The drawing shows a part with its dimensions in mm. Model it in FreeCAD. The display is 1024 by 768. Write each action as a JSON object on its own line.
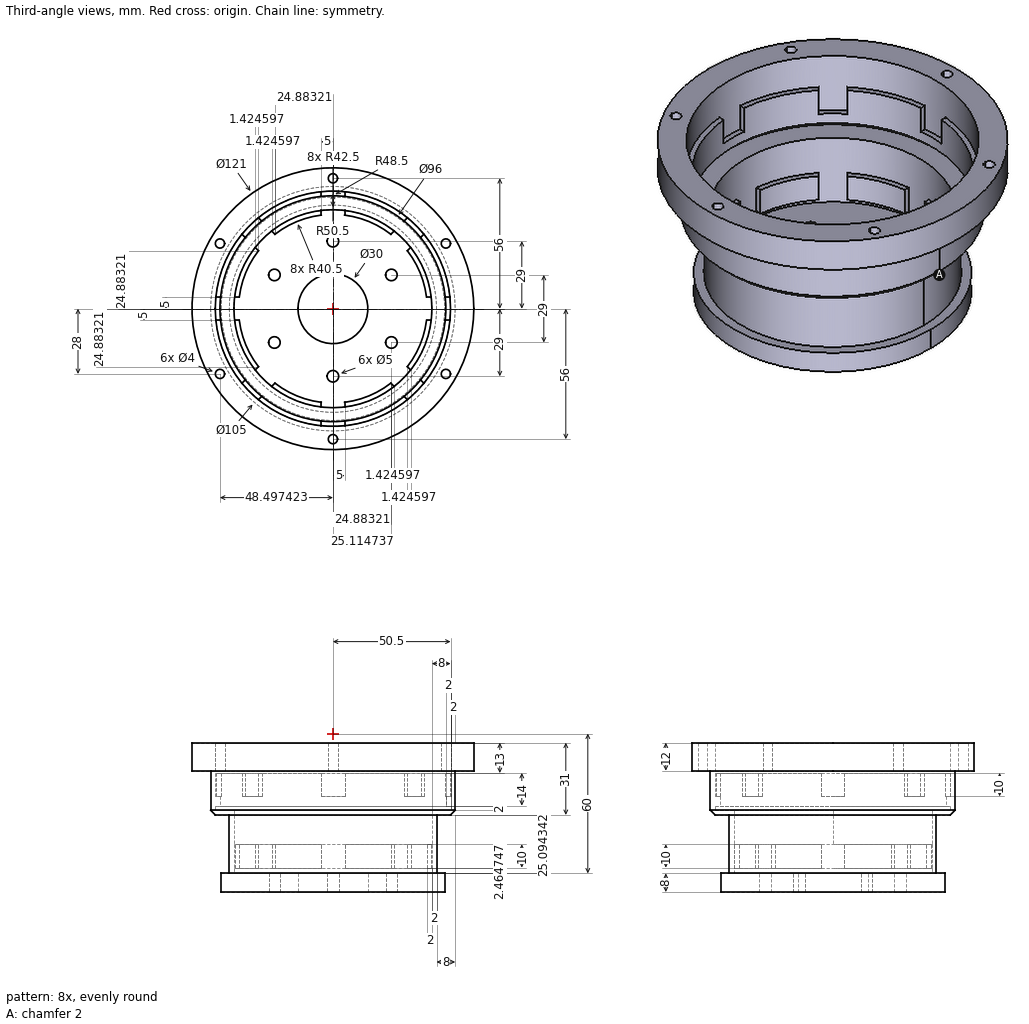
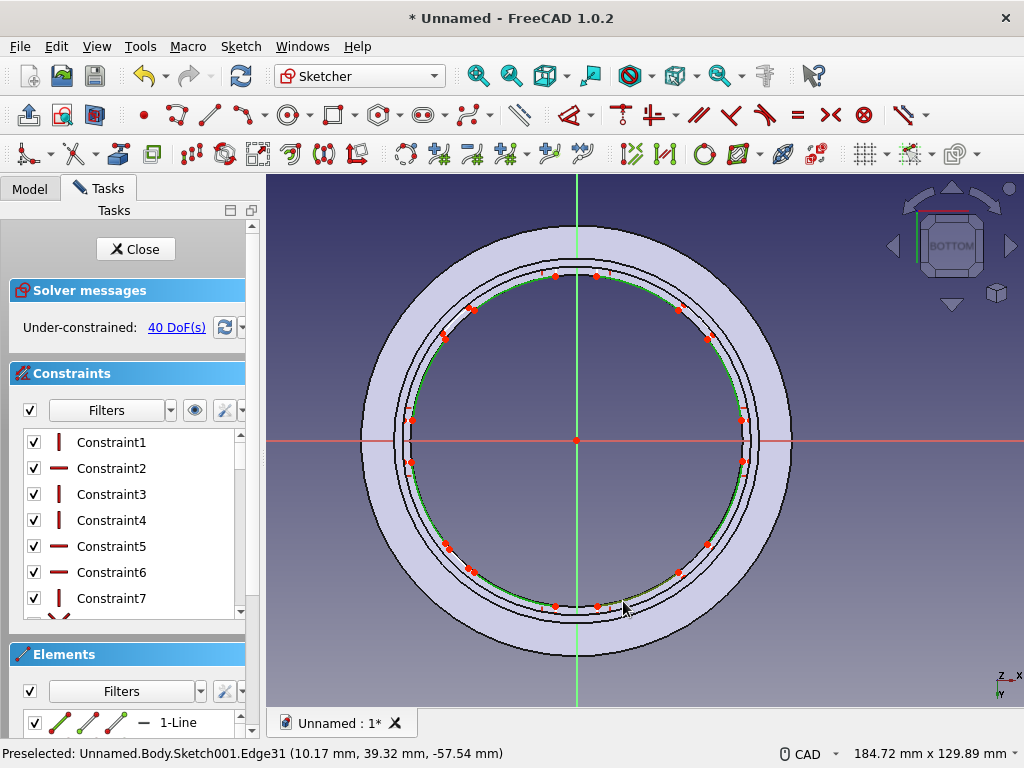
{"action": "left_click", "coordinate": [798, 116]}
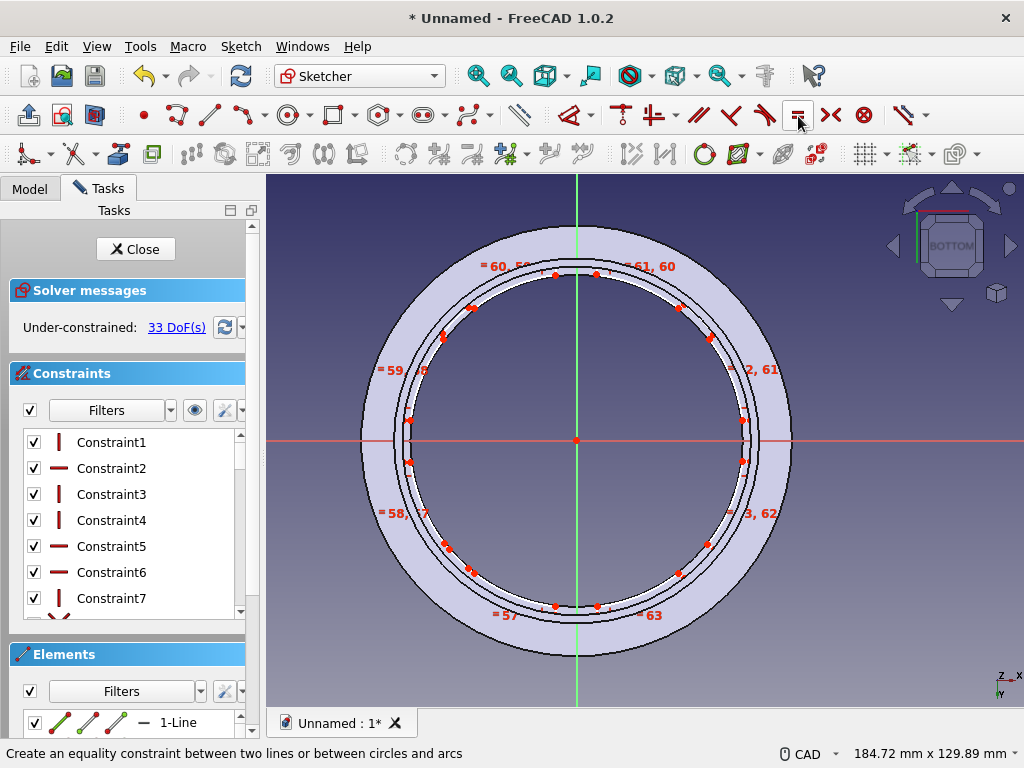
{"action": "left_click", "coordinate": [458, 559]}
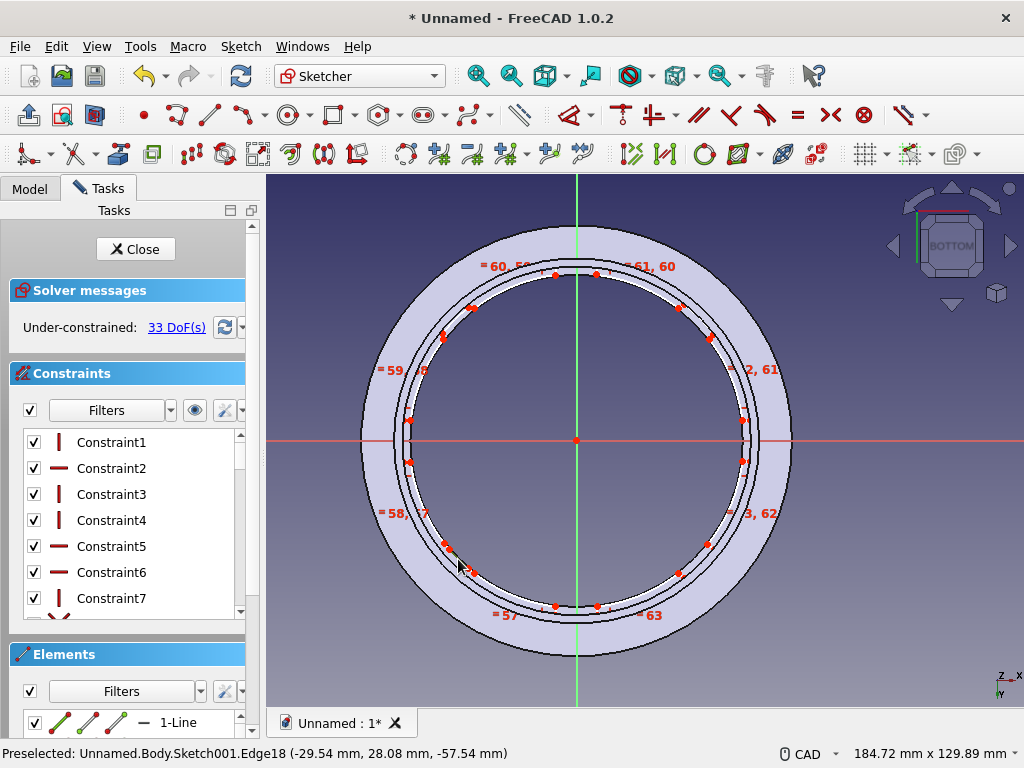
{"action": "scroll", "coordinate": [460, 315], "scroll_direction": "up", "scroll_amount": 2}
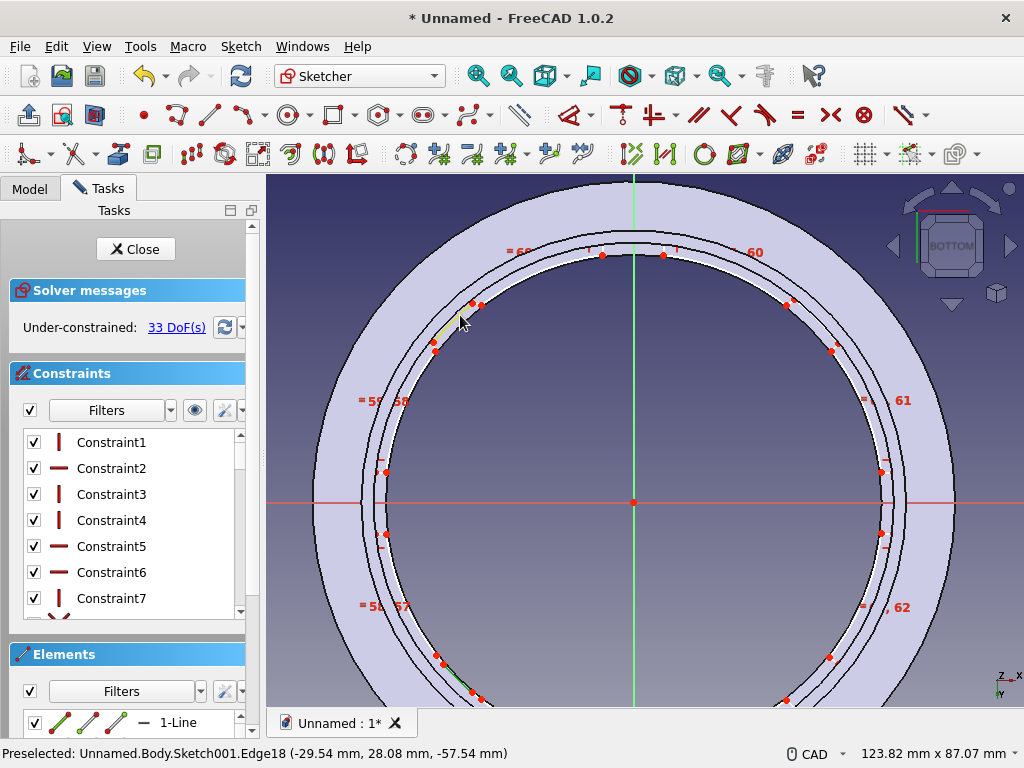
{"action": "left_click", "coordinate": [460, 314]}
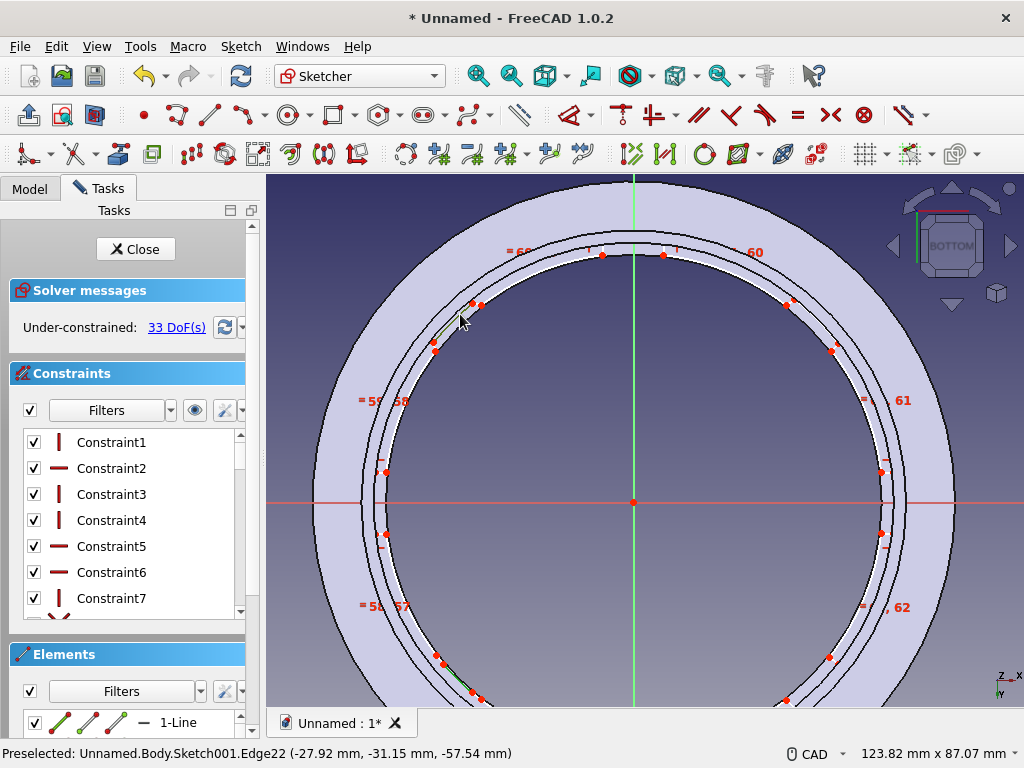
{"action": "left_click", "coordinate": [826, 330]}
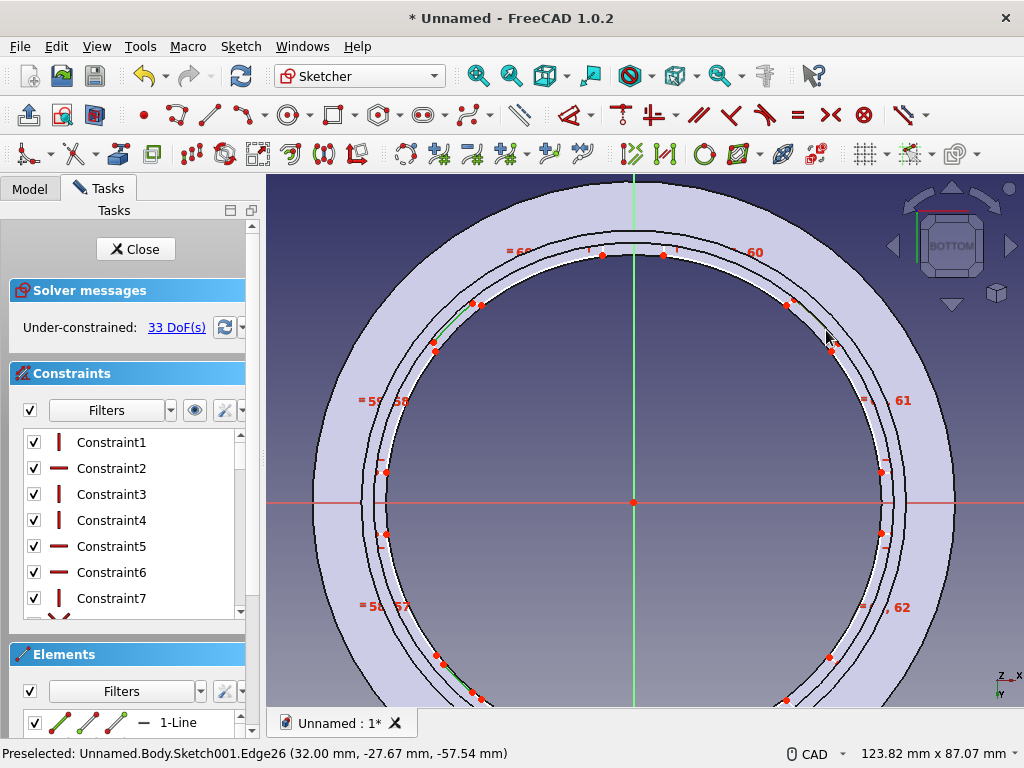
{"action": "left_click", "coordinate": [827, 679]}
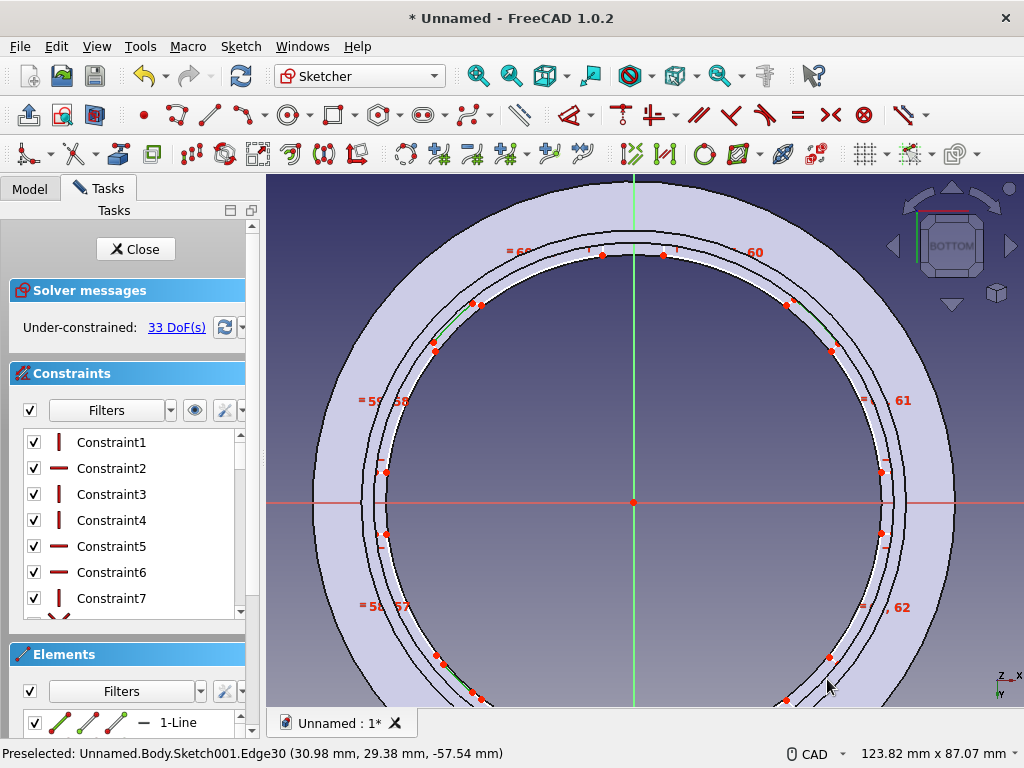
{"action": "key", "text": "e"}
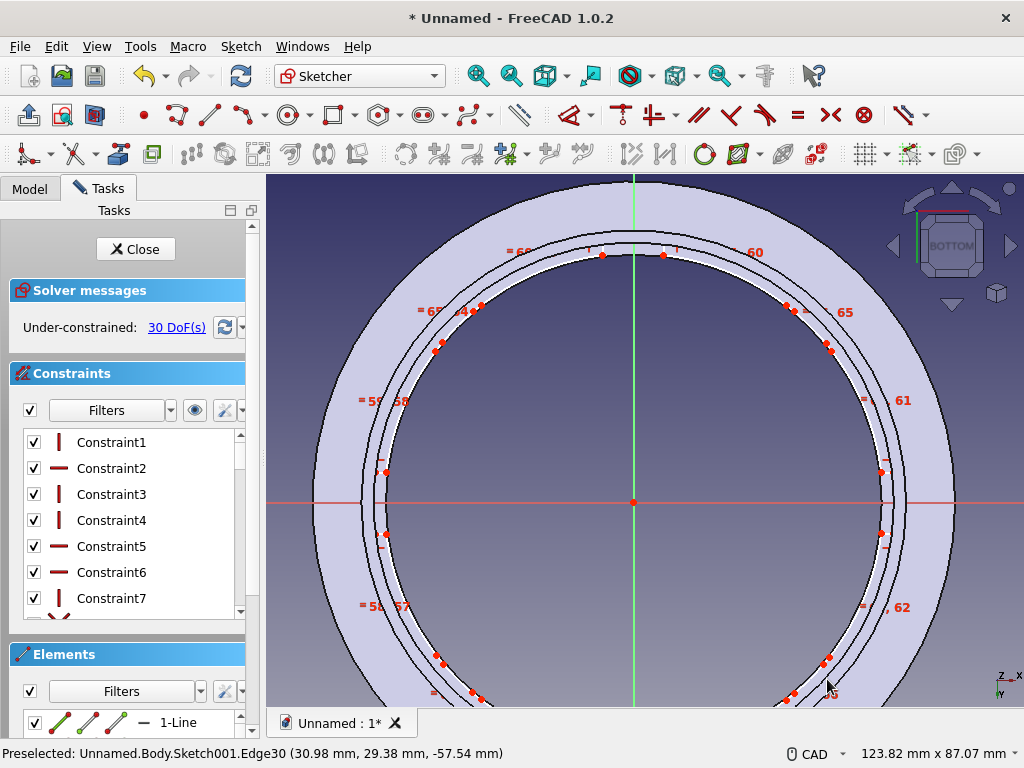
{"action": "left_click", "coordinate": [374, 491]}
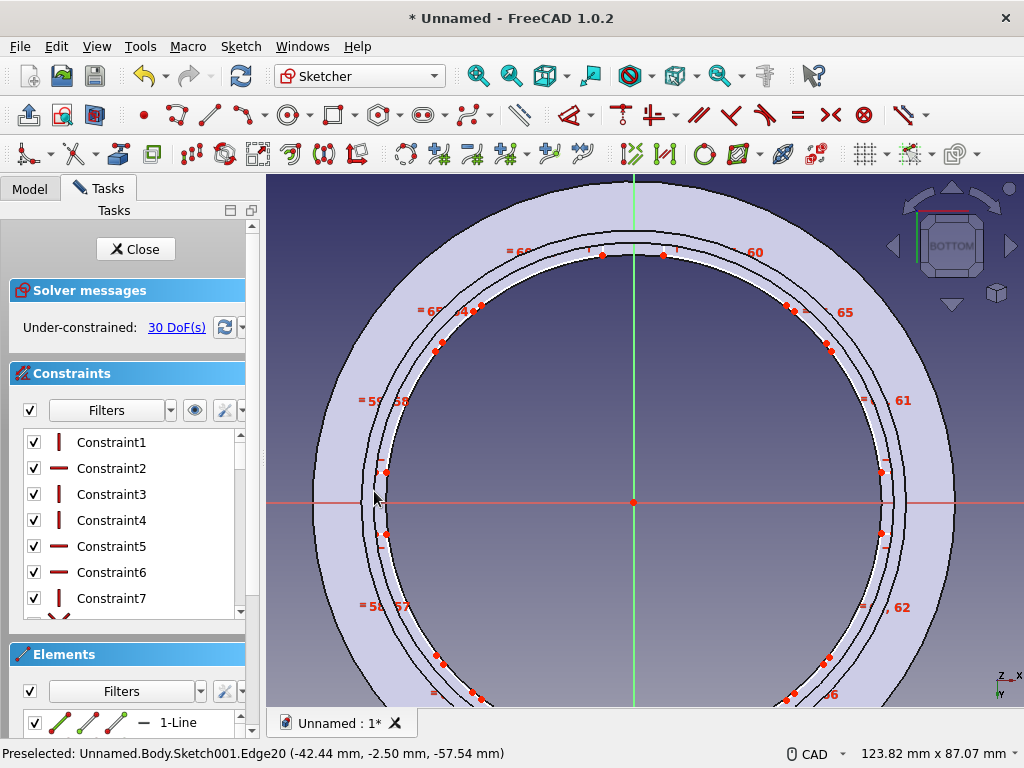
{"action": "left_click", "coordinate": [646, 238]}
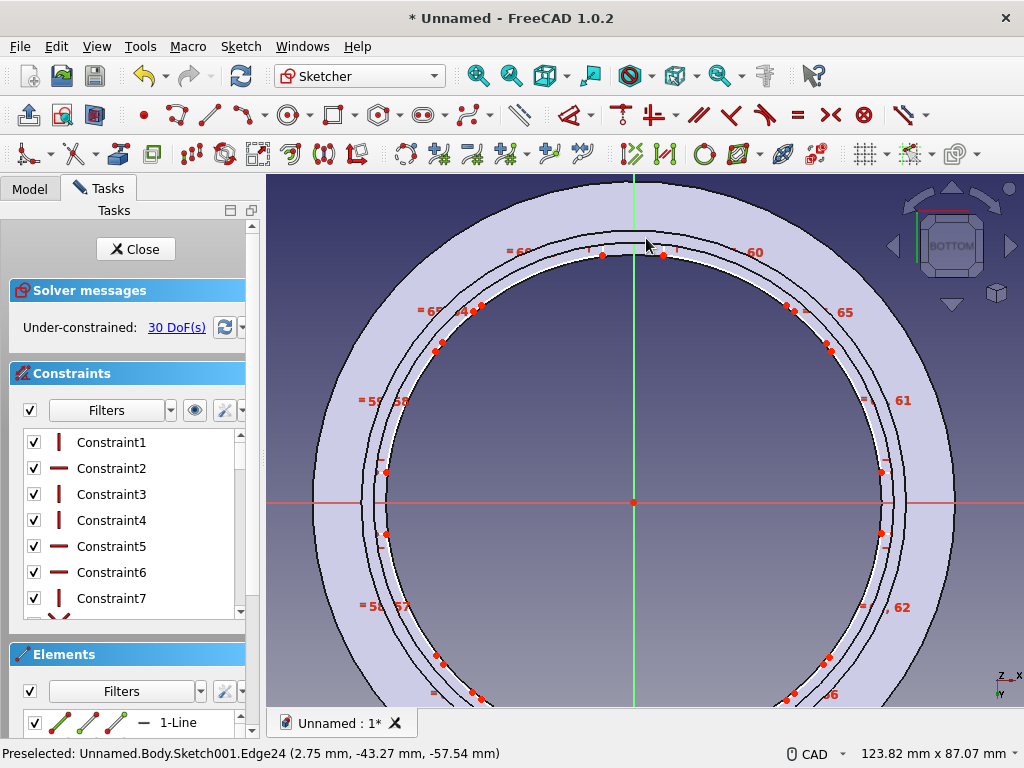
{"action": "scroll", "coordinate": [460, 314], "scroll_direction": "down", "scroll_amount": 2}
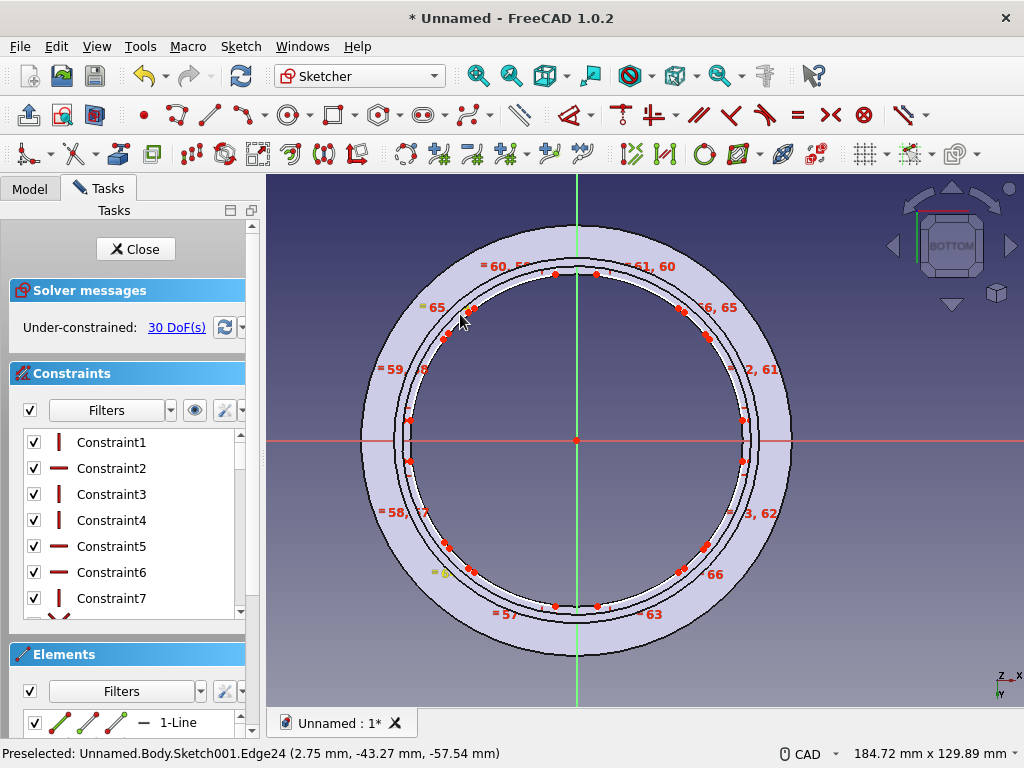
{"action": "scroll", "coordinate": [568, 616], "scroll_direction": "up", "scroll_amount": 3}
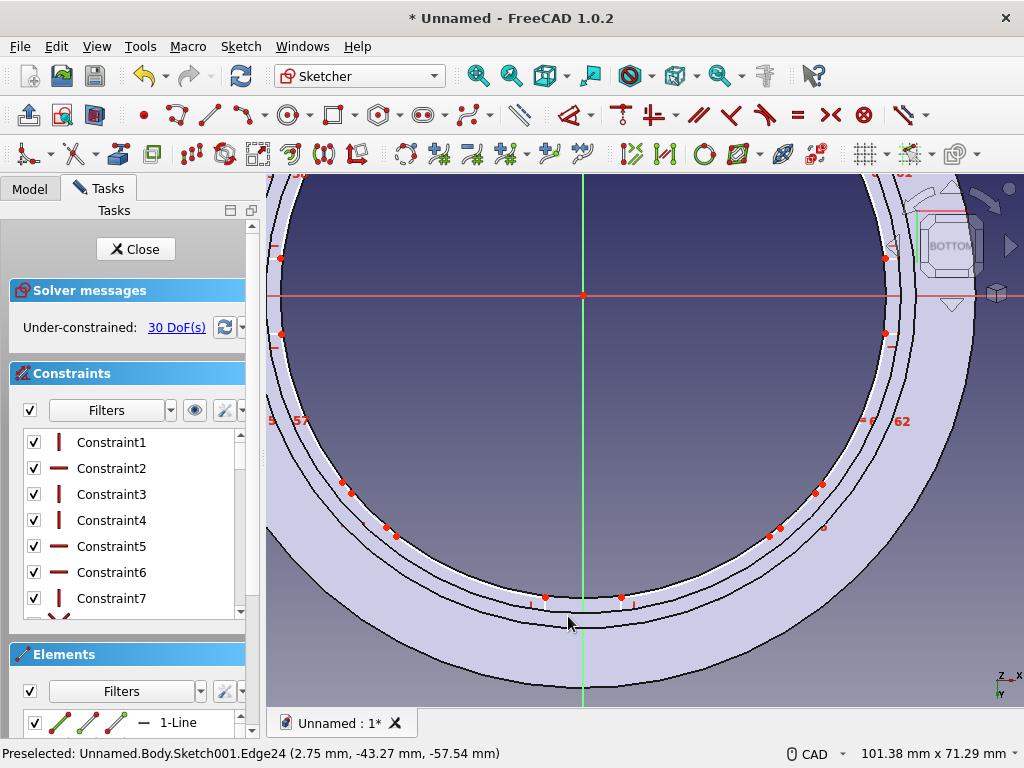
{"action": "left_click", "coordinate": [568, 616]}